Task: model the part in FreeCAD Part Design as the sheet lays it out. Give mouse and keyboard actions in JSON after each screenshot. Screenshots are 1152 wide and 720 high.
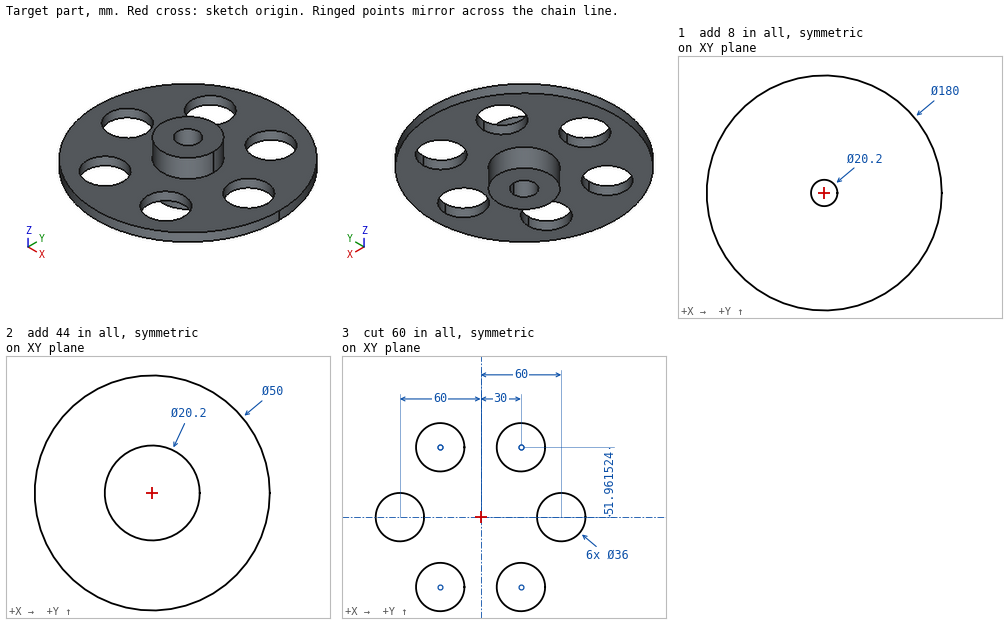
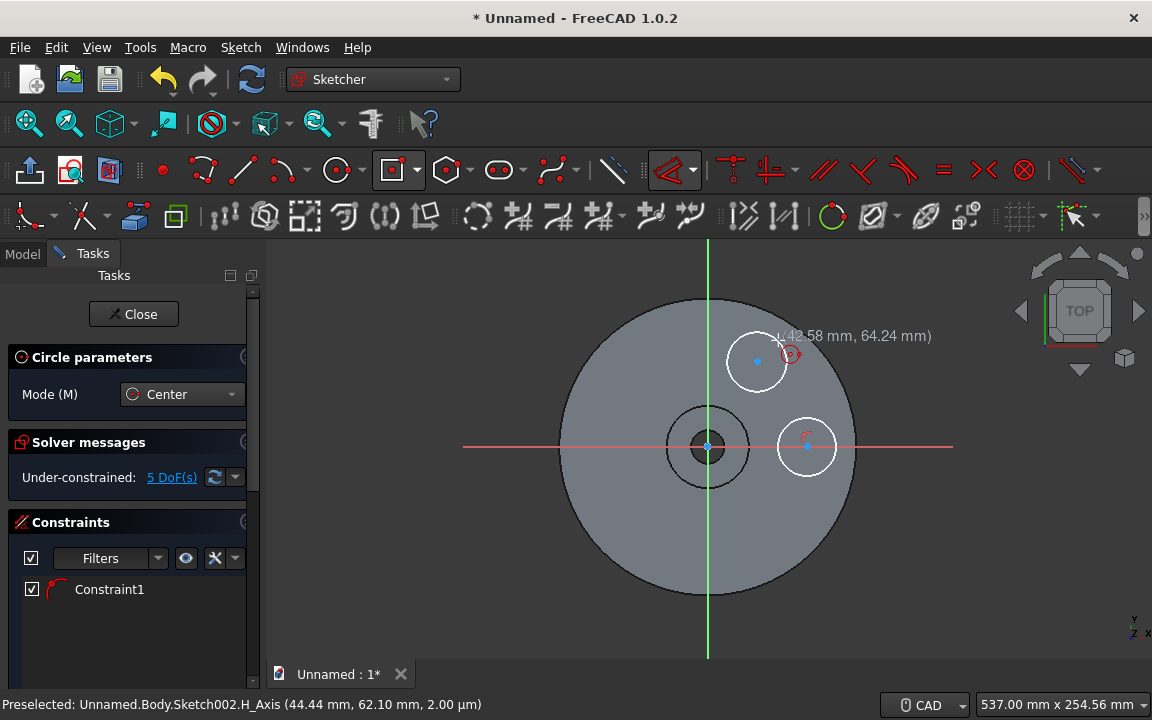
{"action": "left_click", "coordinate": [658, 361]}
{"action": "left_click", "coordinate": [679, 340]}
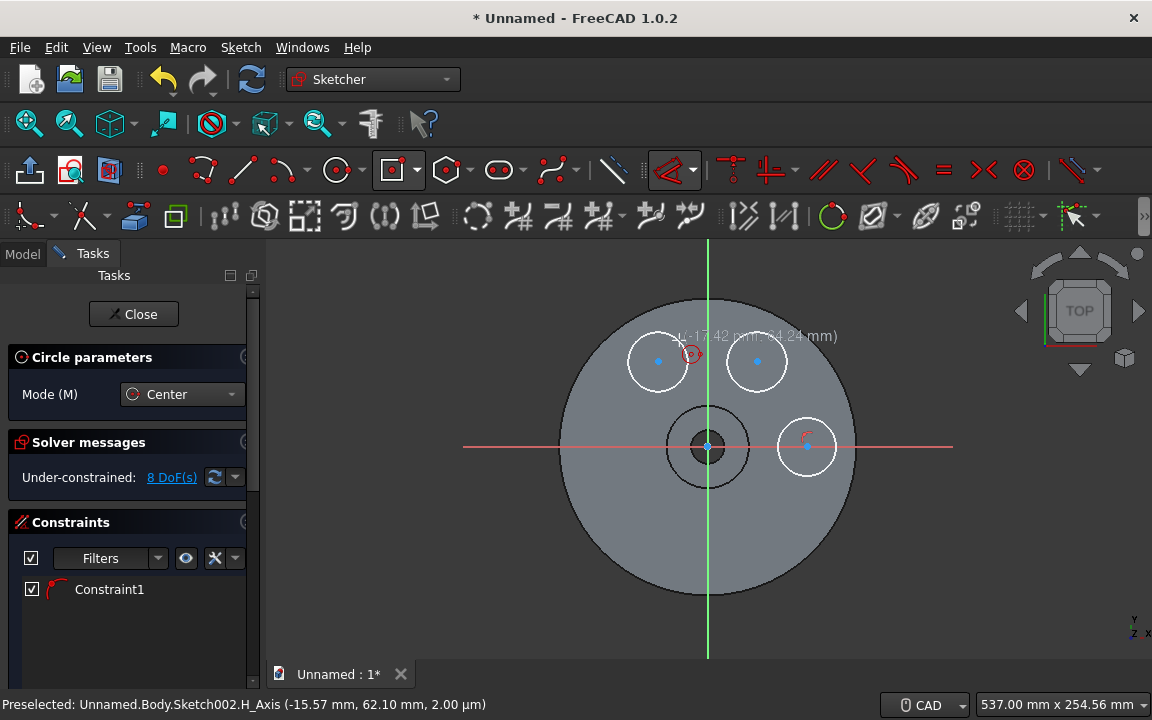
{"action": "left_click", "coordinate": [609, 447]}
{"action": "left_click", "coordinate": [630, 426]}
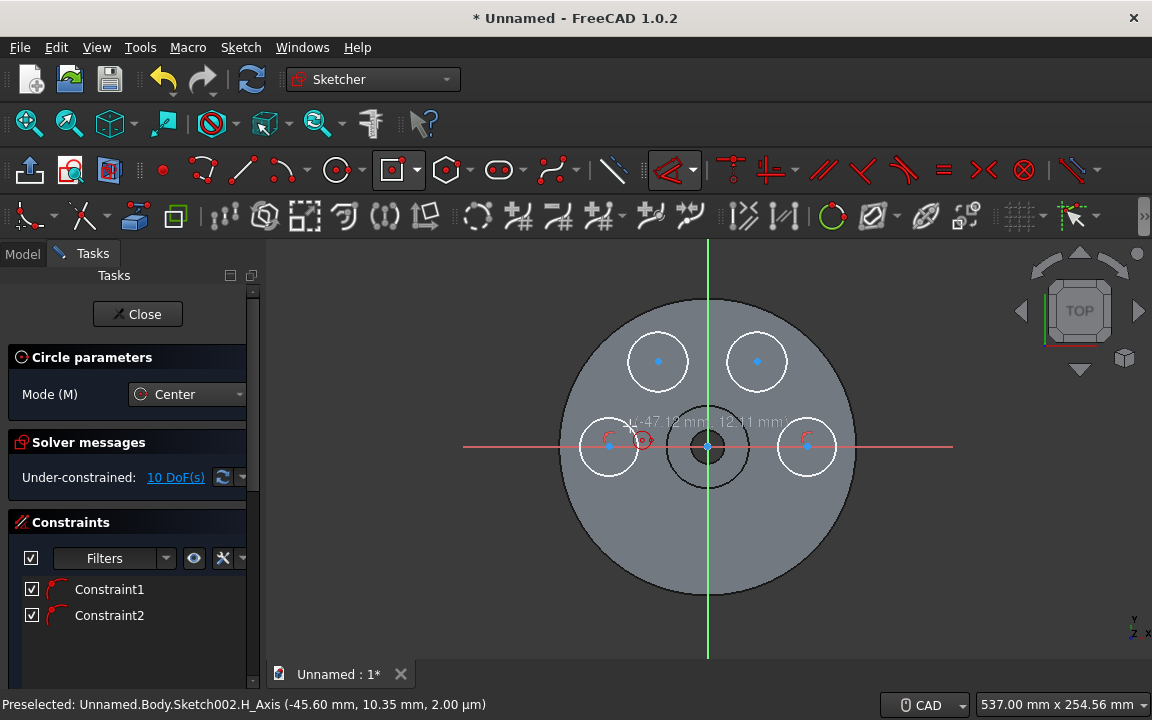
{"action": "left_click", "coordinate": [658, 533]}
{"action": "left_click", "coordinate": [679, 512]}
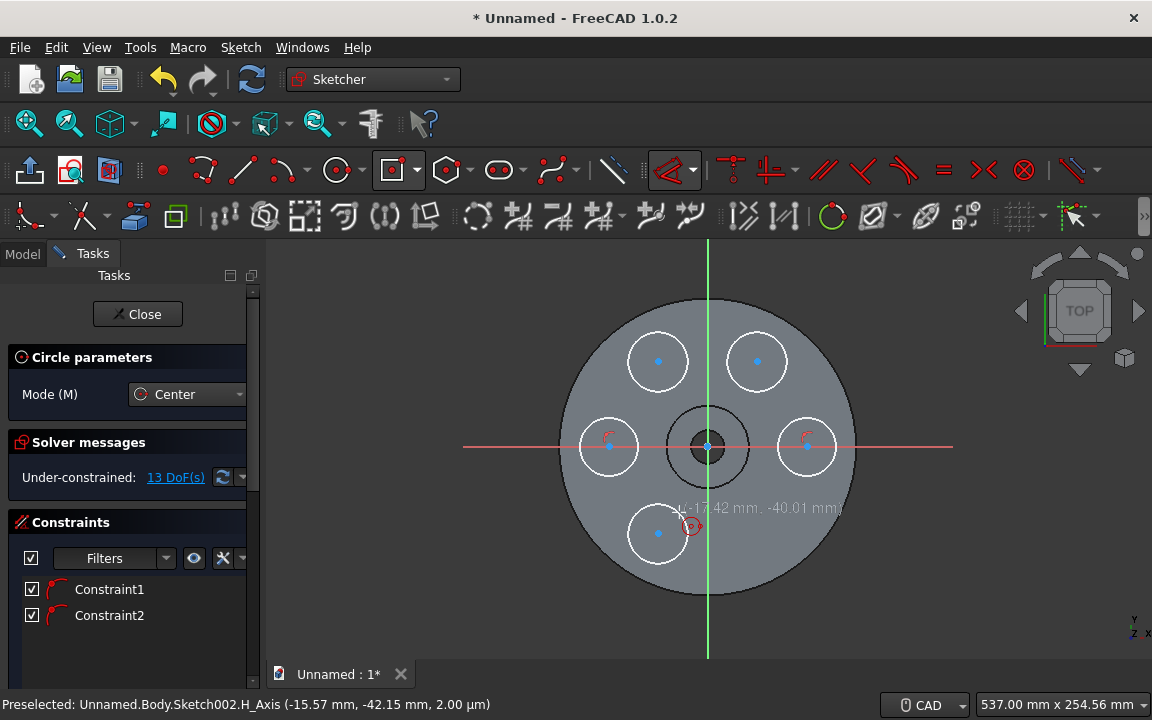
{"action": "left_click", "coordinate": [757, 533]}
{"action": "left_click", "coordinate": [778, 512]}
{"action": "key", "text": "Escape"}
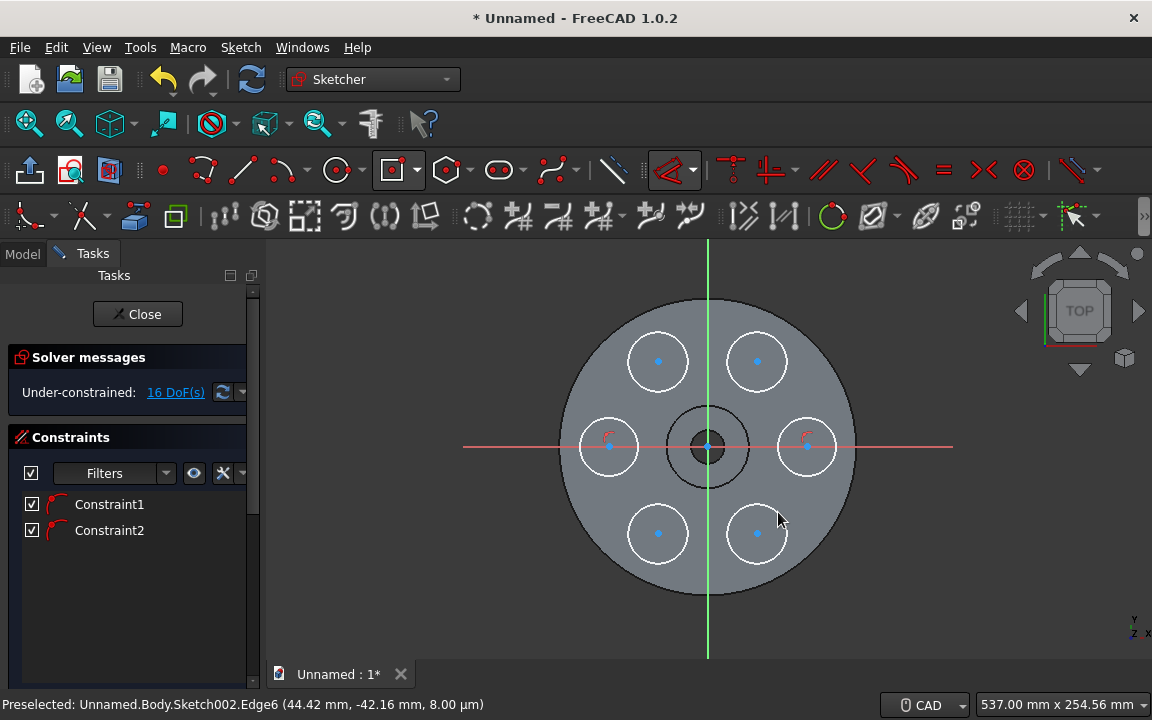
{"action": "left_click", "coordinate": [827, 426]}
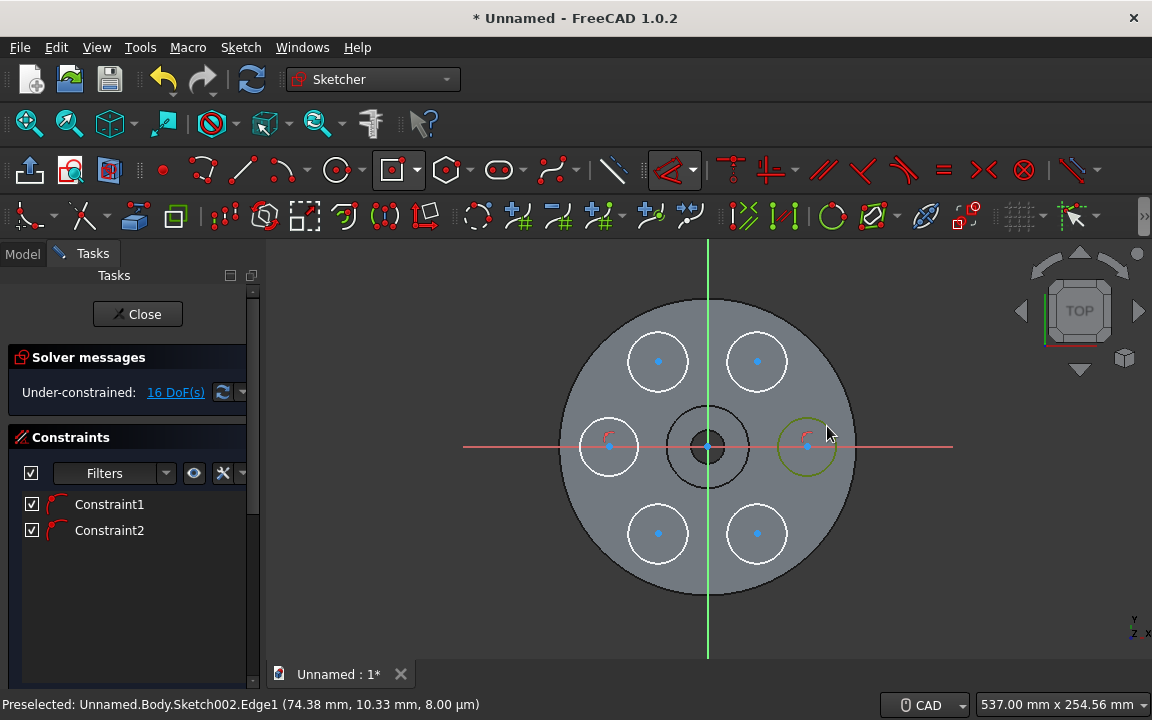
{"action": "left_click", "coordinate": [778, 341]}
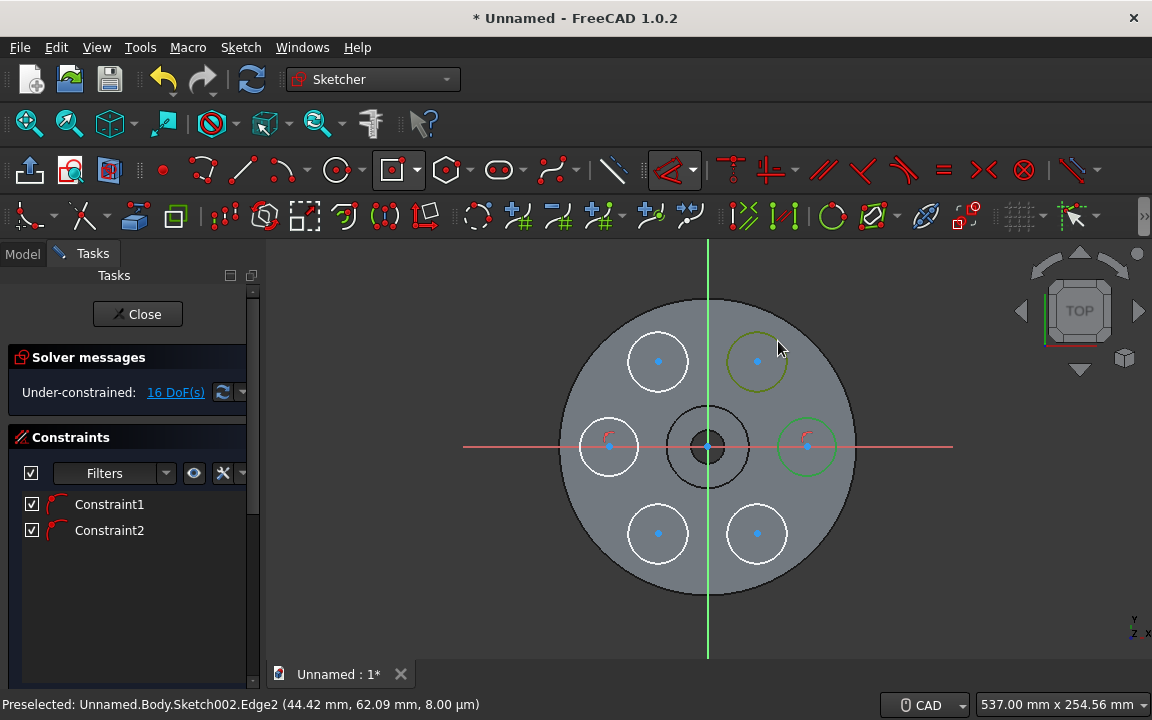
{"action": "left_click", "coordinate": [679, 341]}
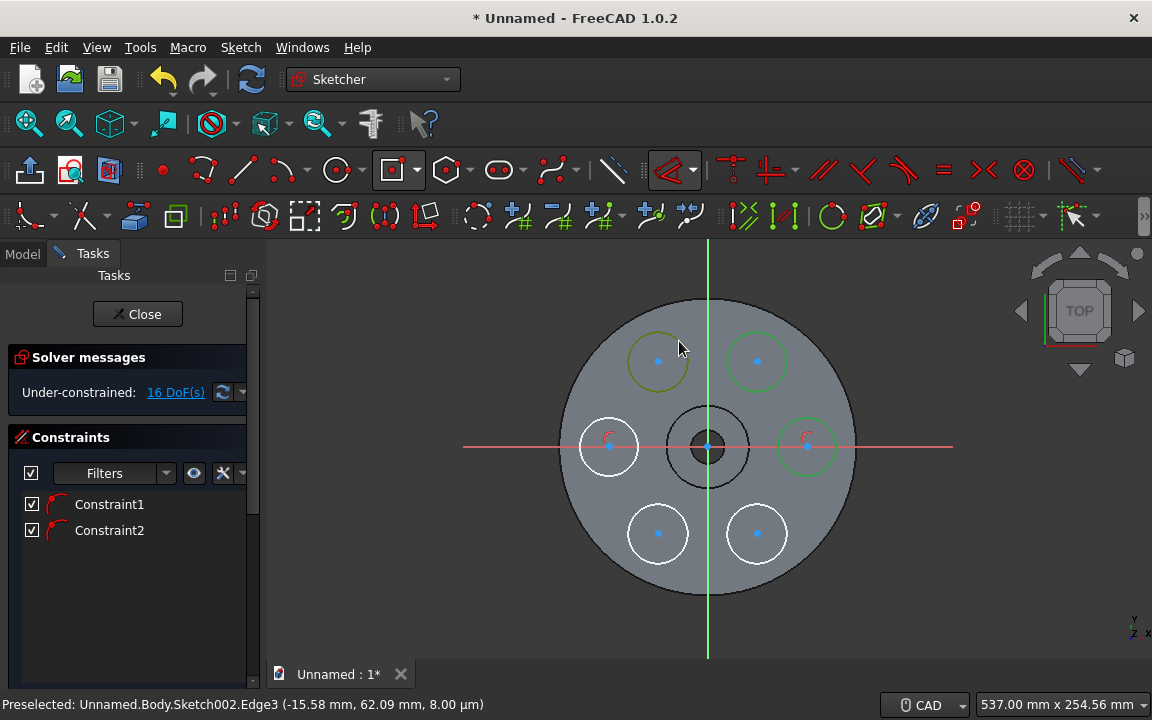
{"action": "left_click", "coordinate": [629, 426]}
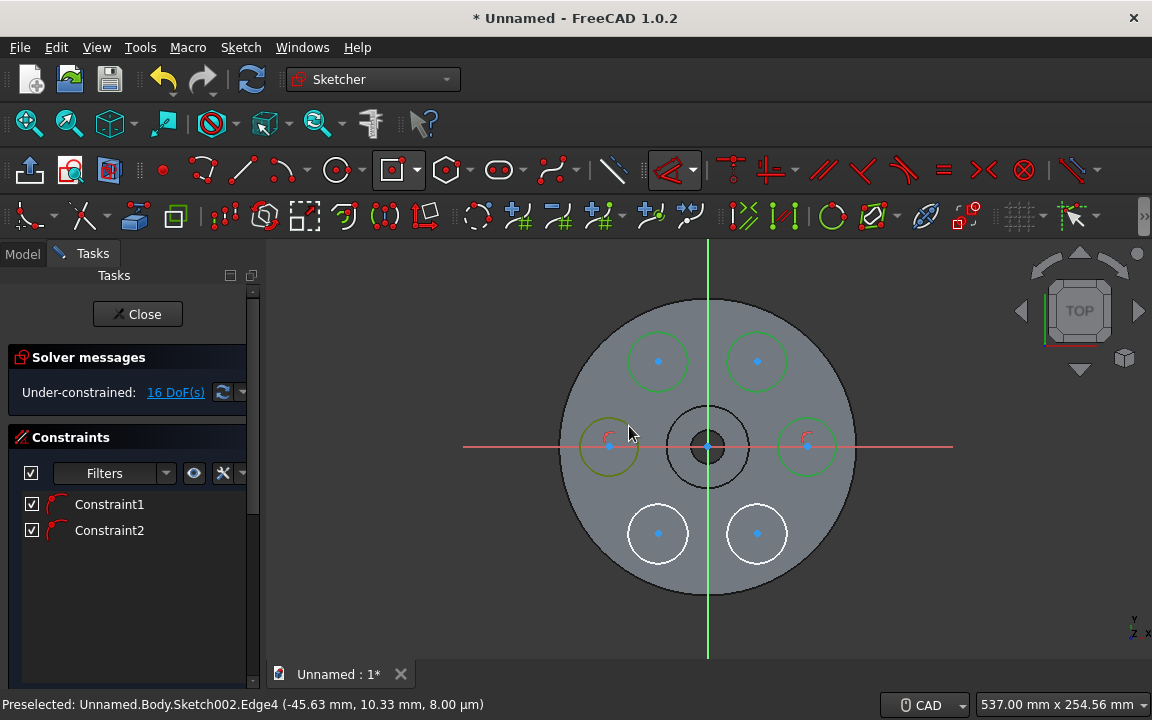
{"action": "left_click", "coordinate": [679, 513]}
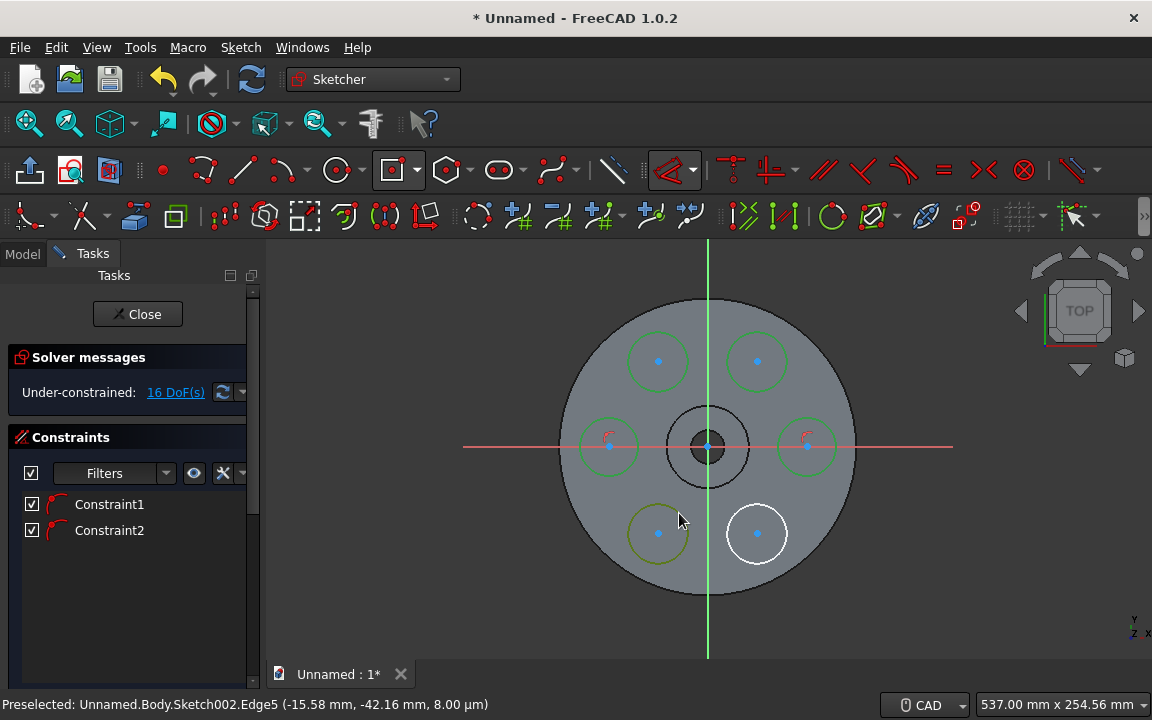
{"action": "left_click", "coordinate": [778, 513]}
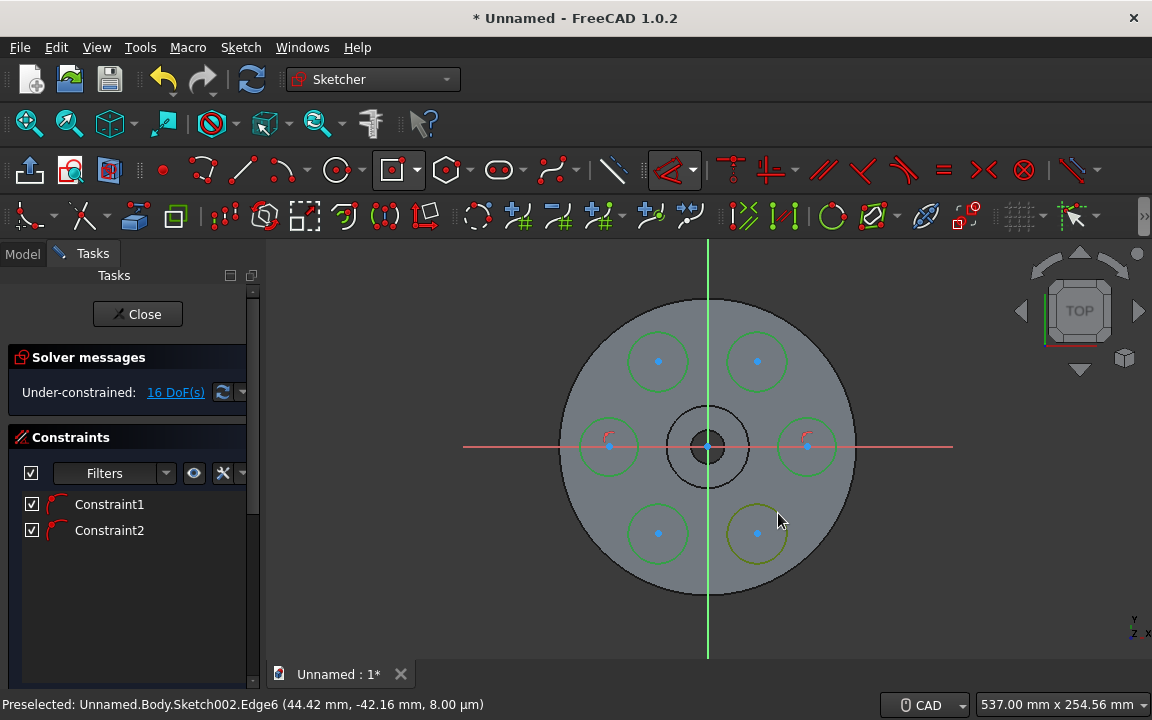
{"action": "left_click", "coordinate": [944, 170]}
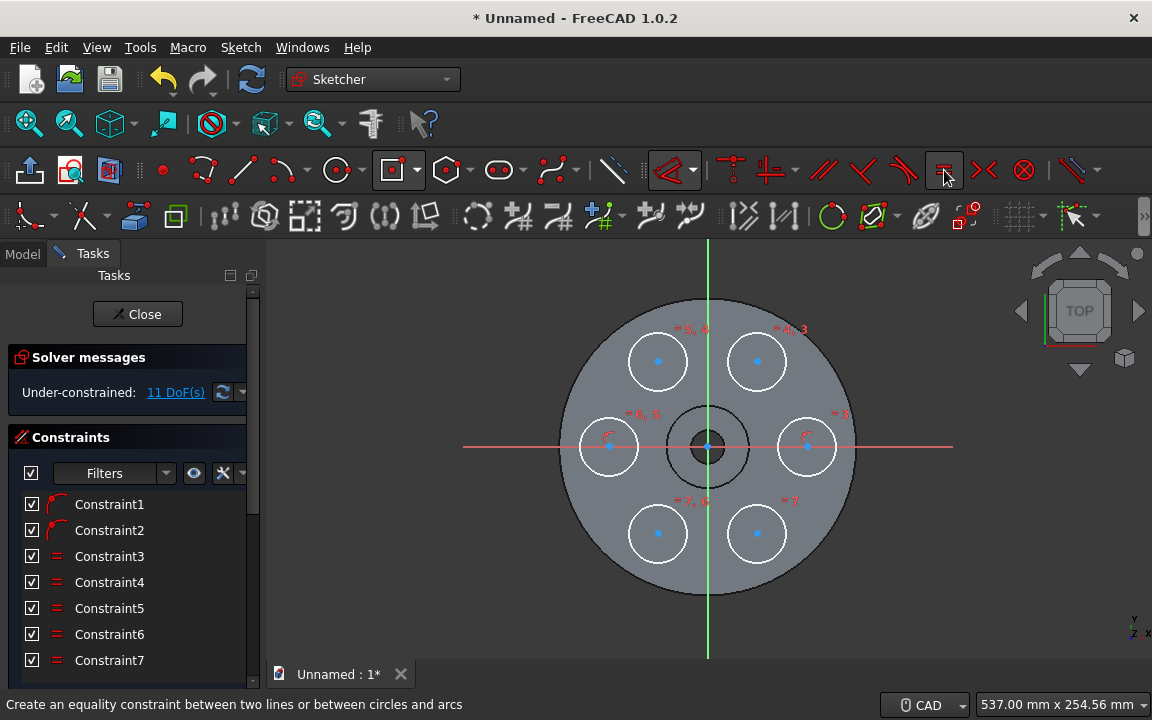
{"action": "left_click", "coordinate": [757, 362]}